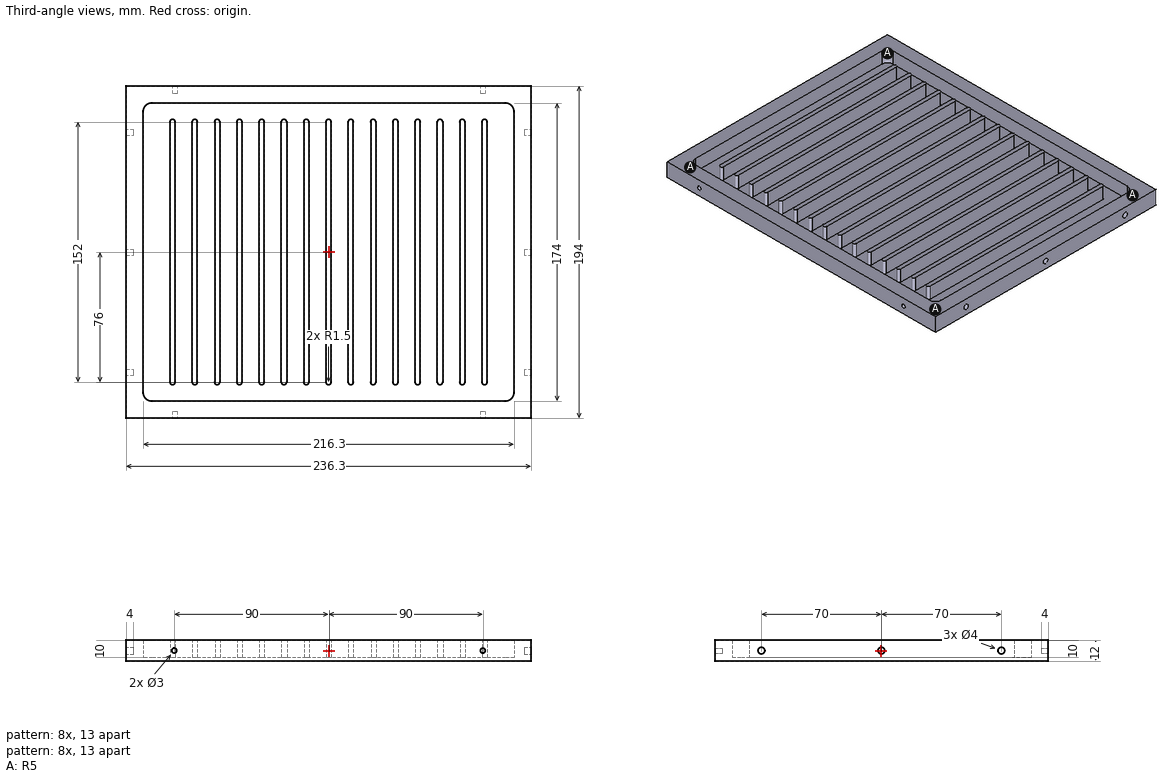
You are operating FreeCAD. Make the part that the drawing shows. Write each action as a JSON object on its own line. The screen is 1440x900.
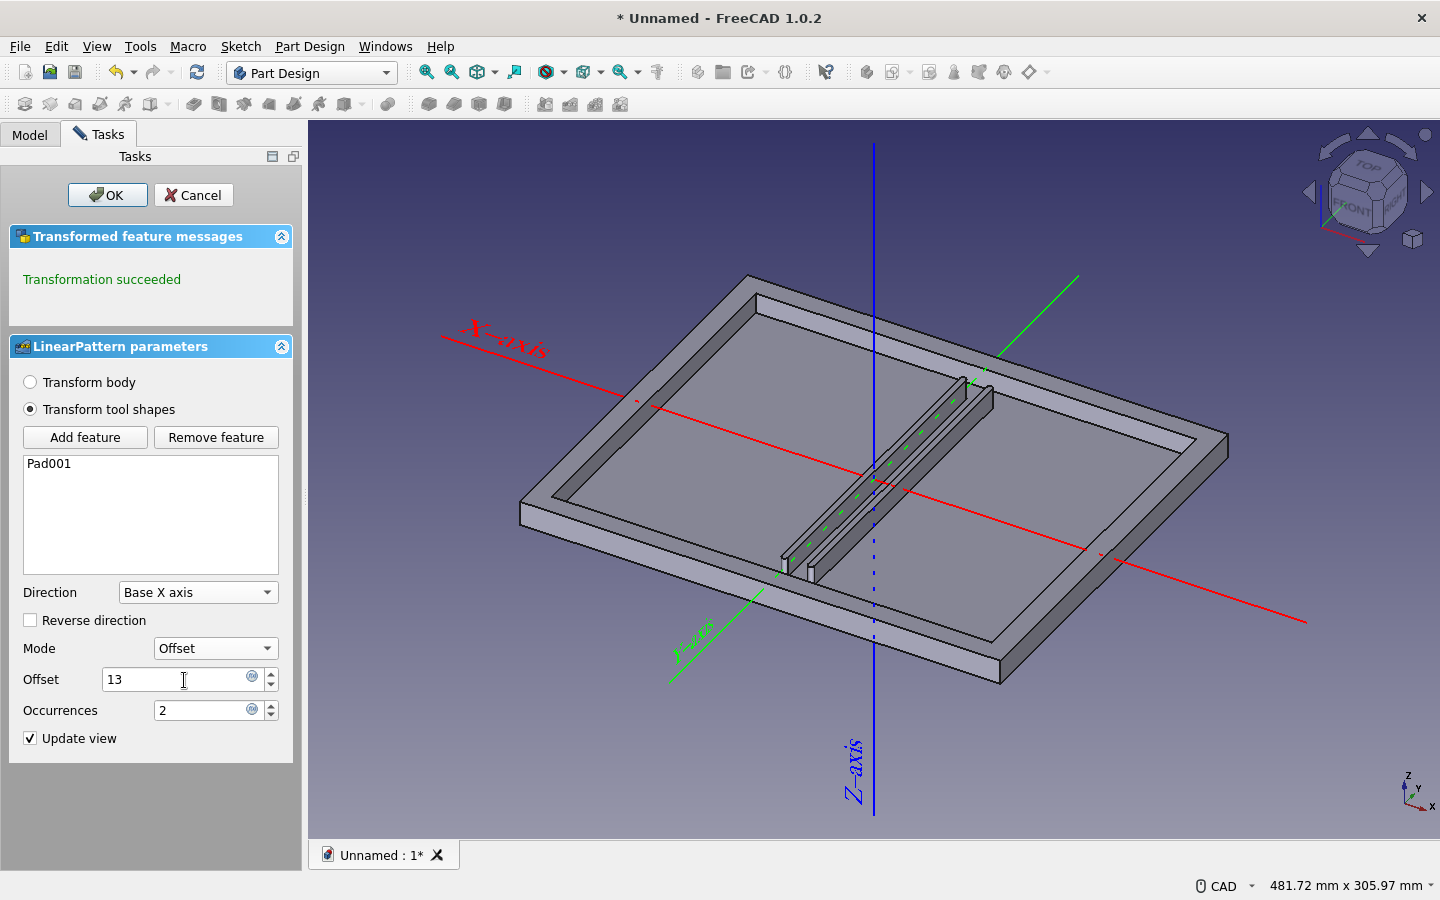
{"action": "triple_click", "coordinate": [210, 710]}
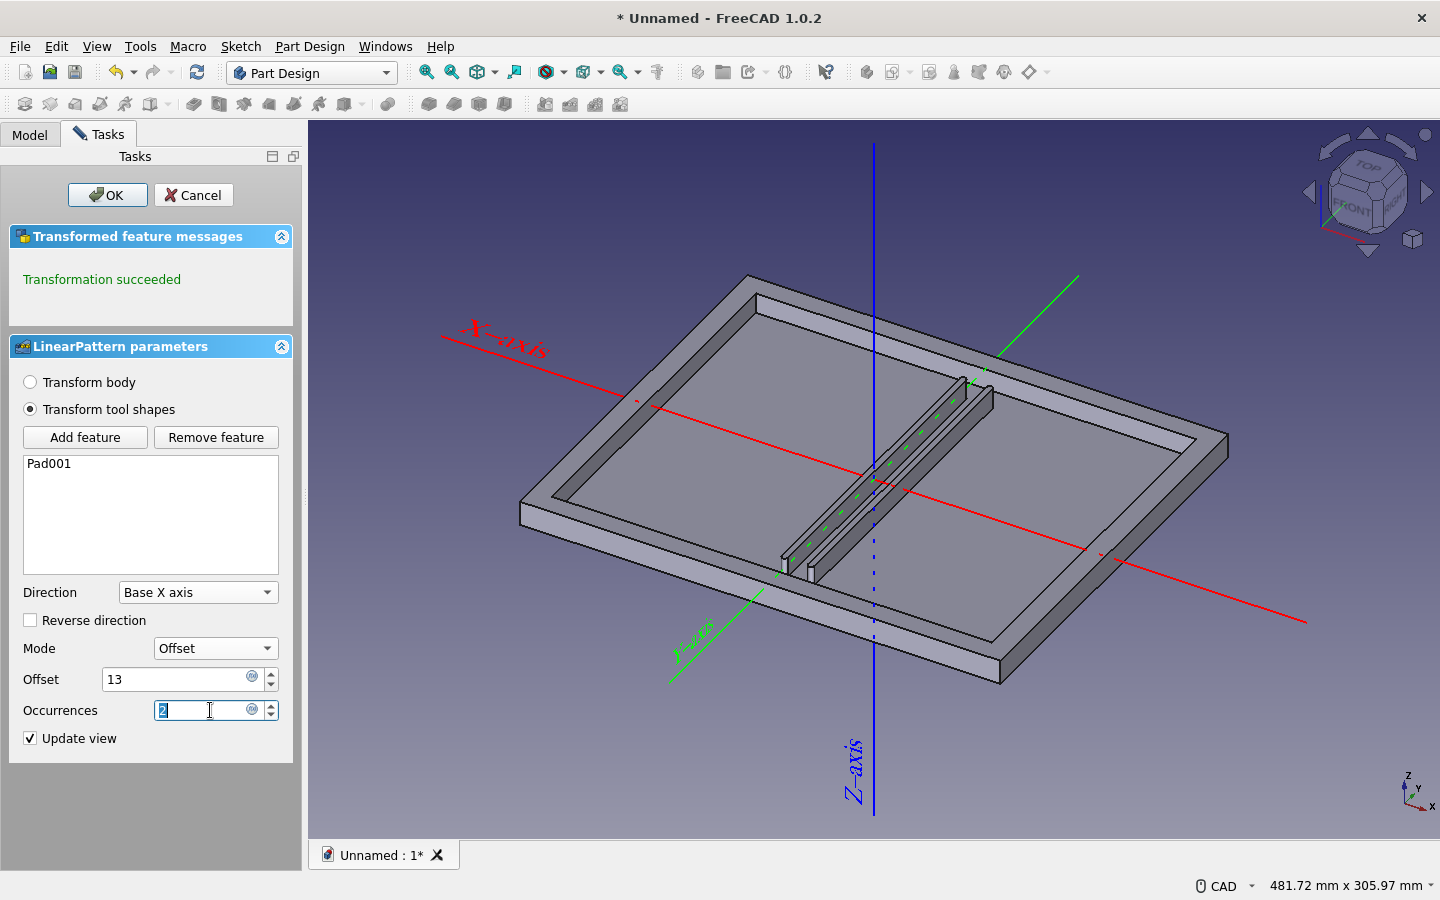
{"action": "type", "text": "8"}
{"action": "key", "text": "Tab"}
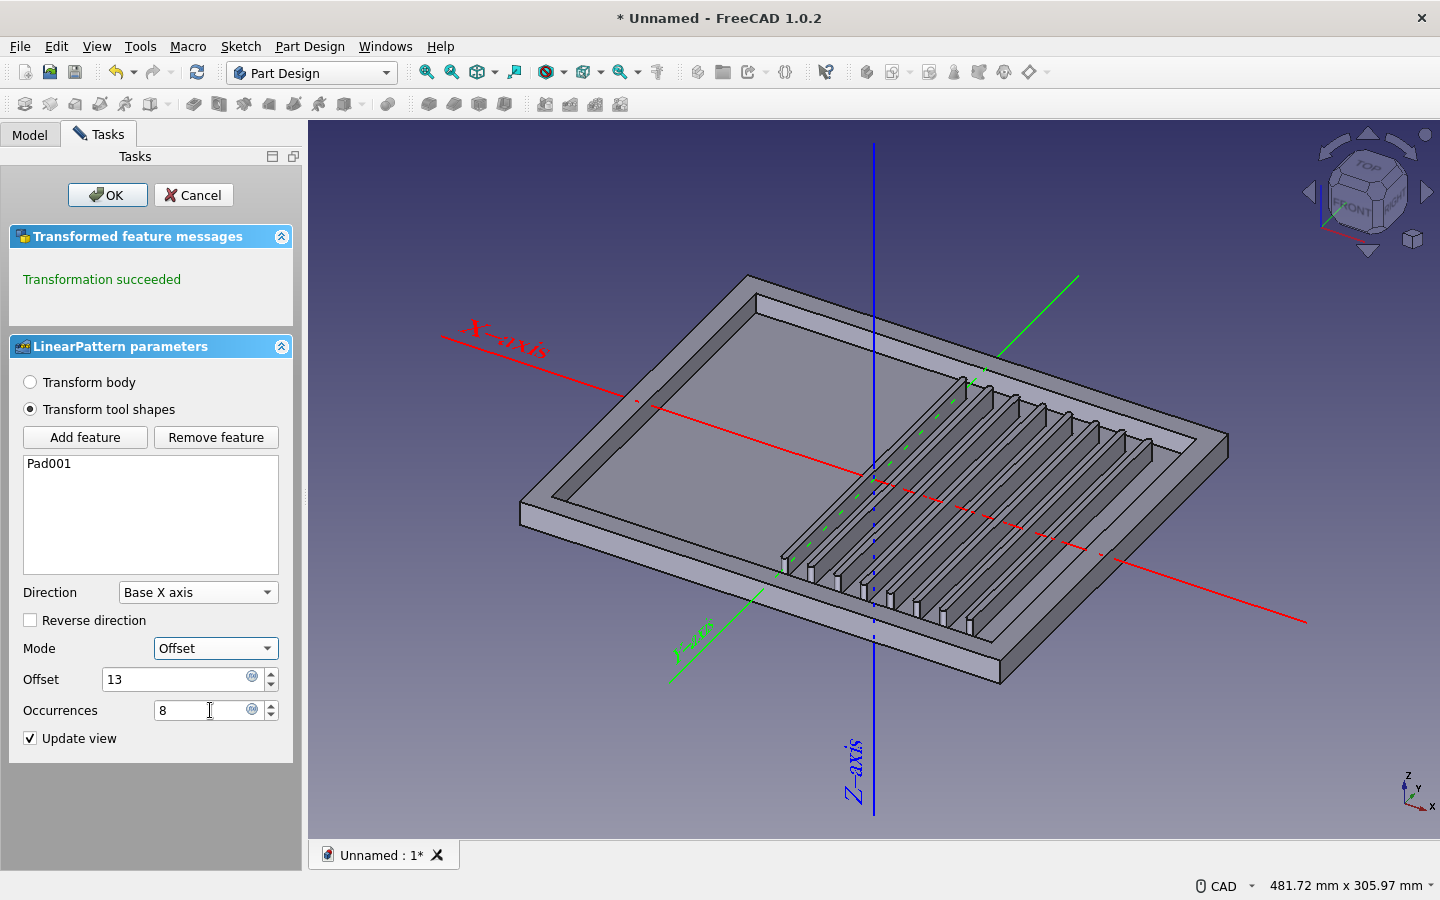
{"action": "left_click", "coordinate": [108, 195]}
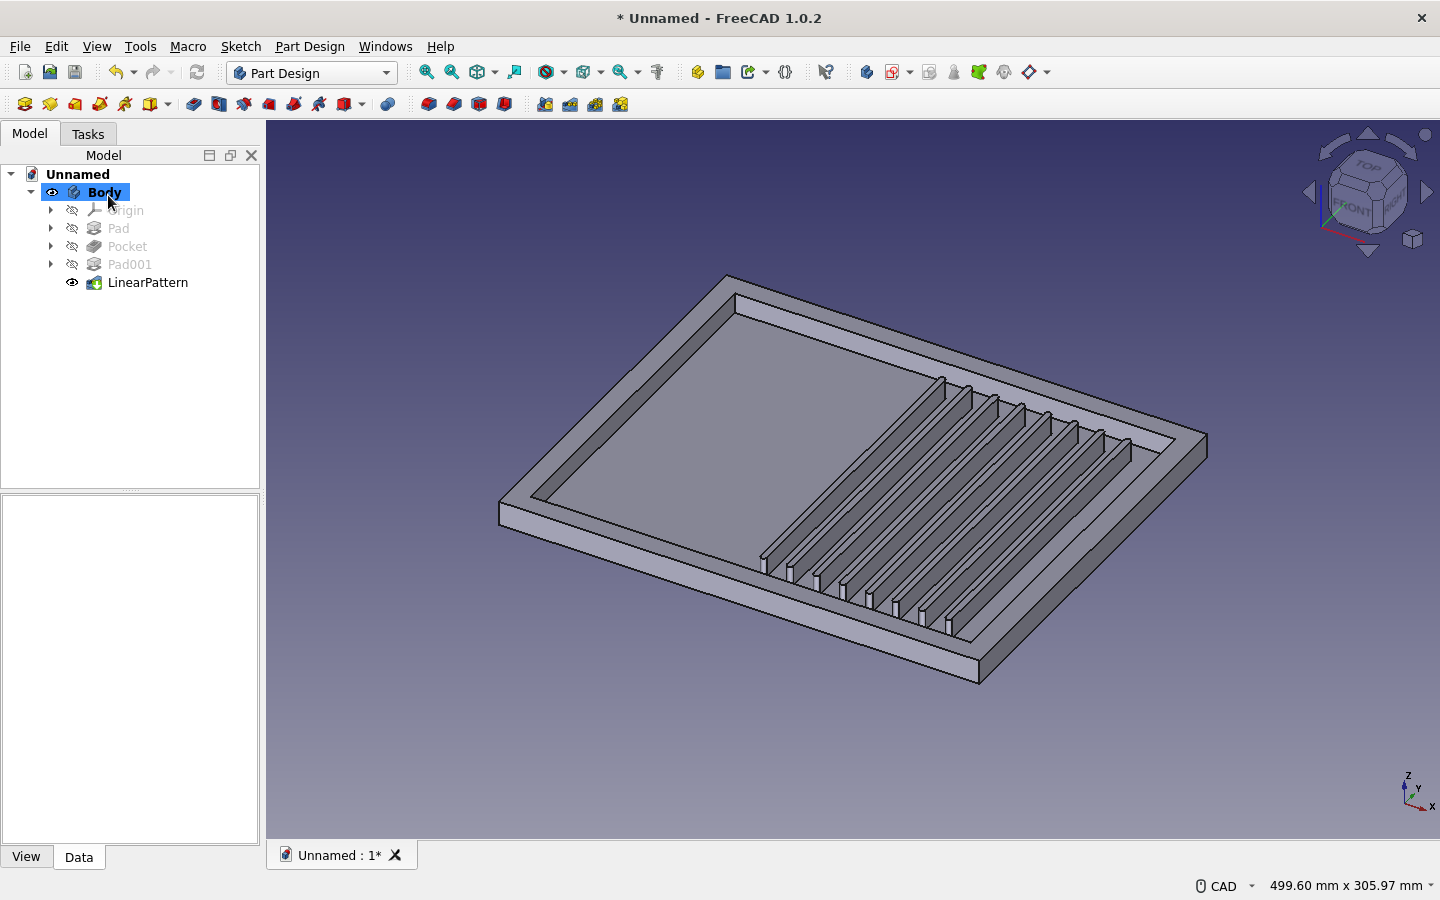
{"action": "left_click", "coordinate": [117, 264]}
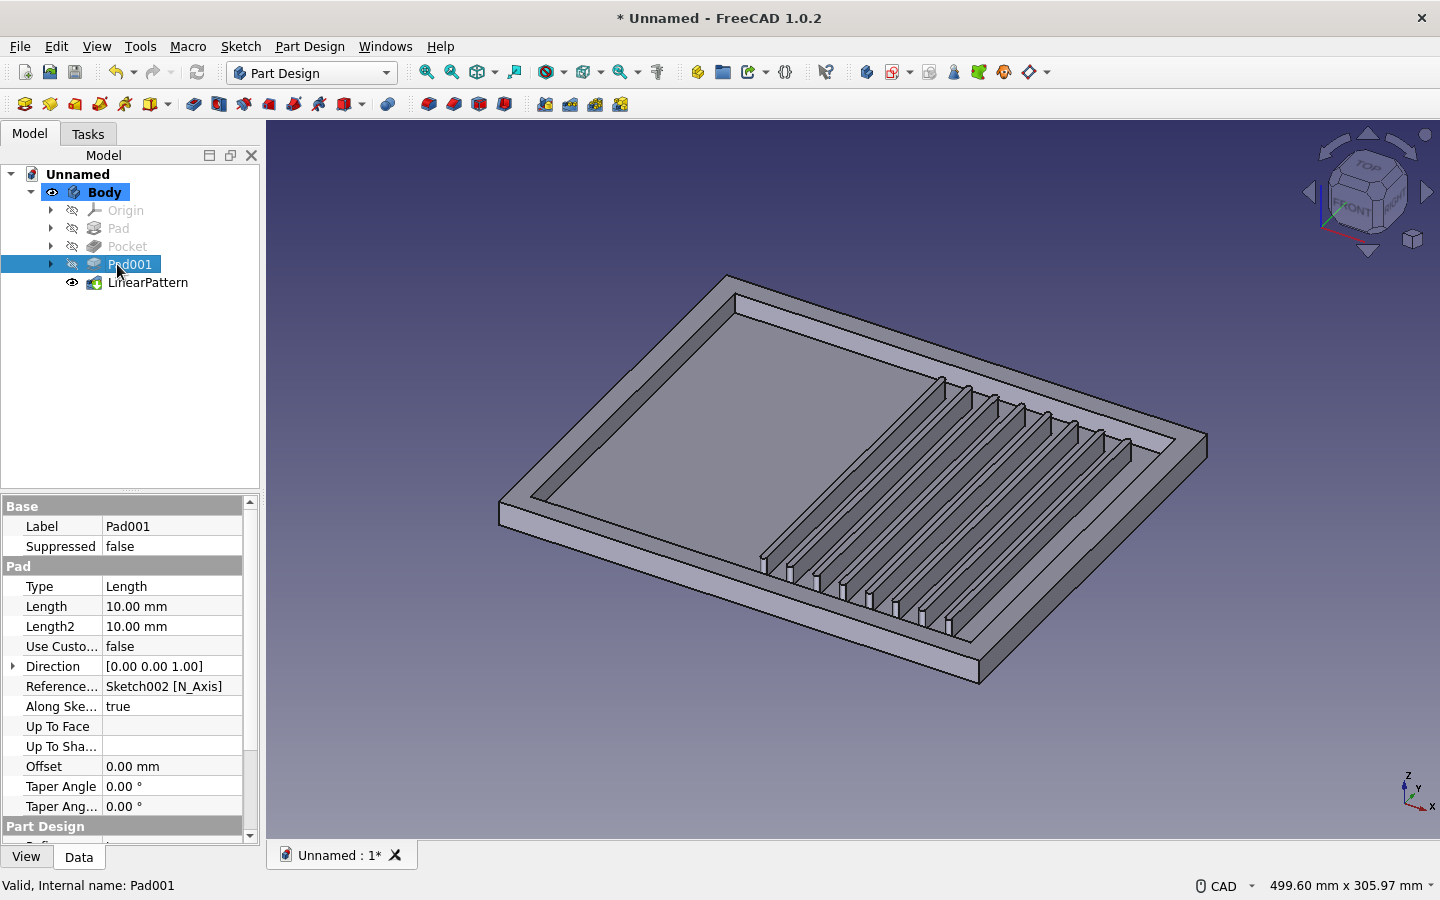
{"action": "left_click", "coordinate": [570, 104]}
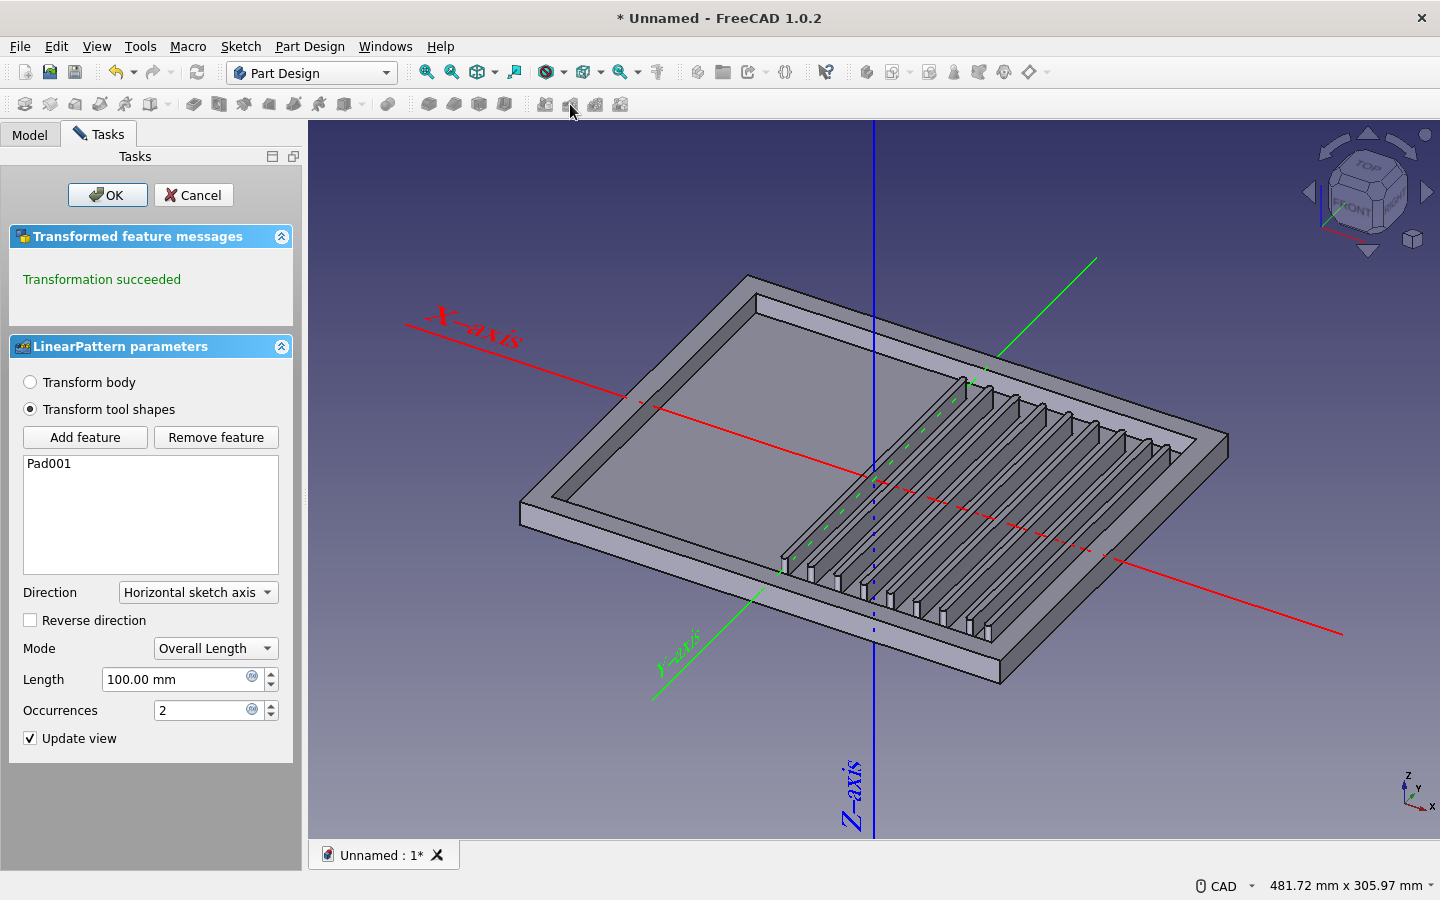
{"action": "left_click", "coordinate": [199, 592]}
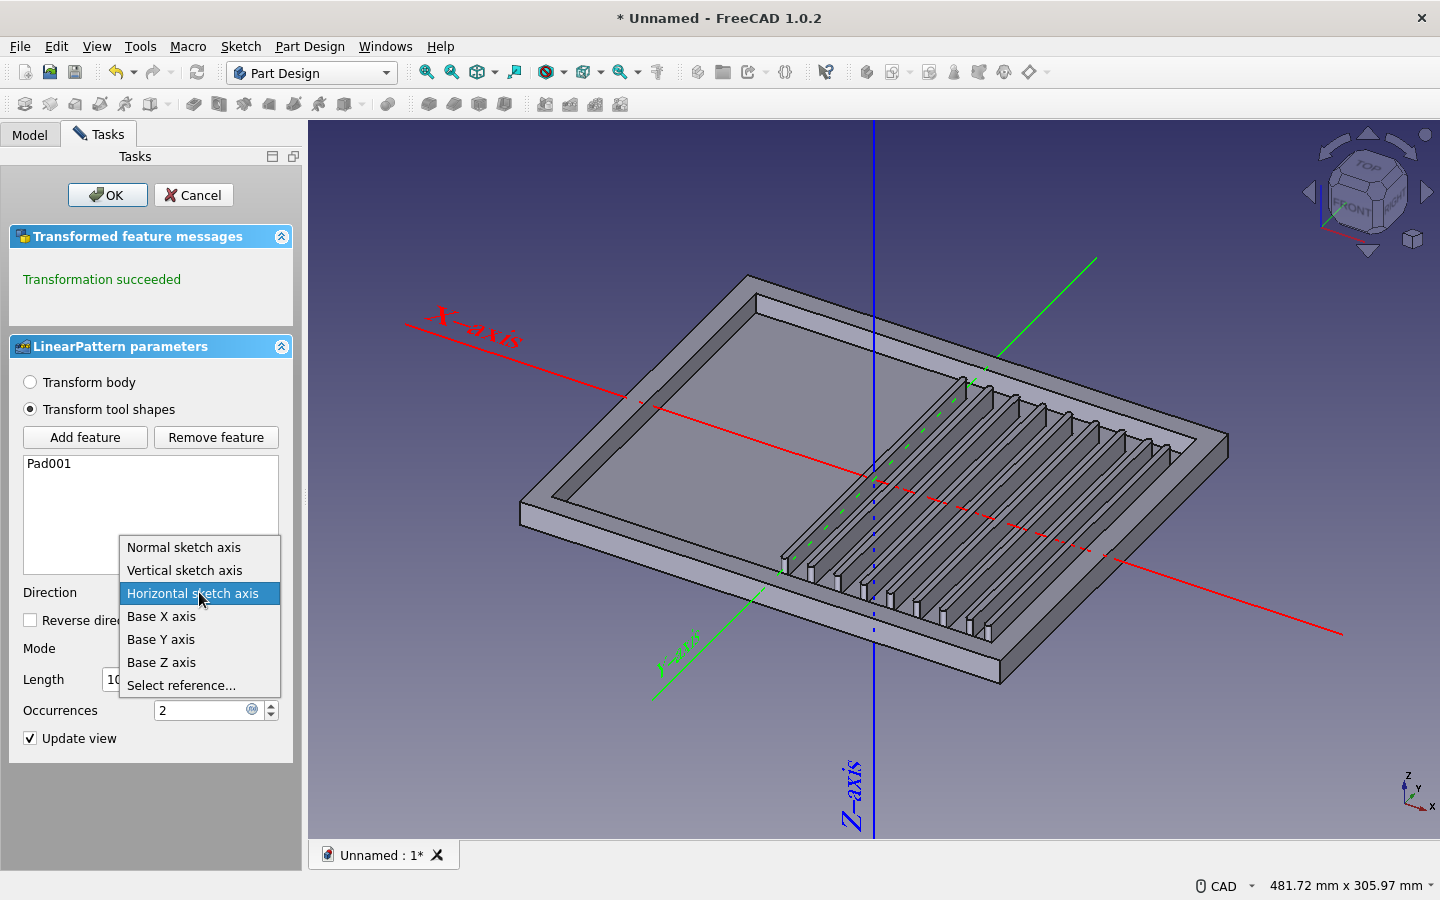
{"action": "left_click", "coordinate": [198, 616]}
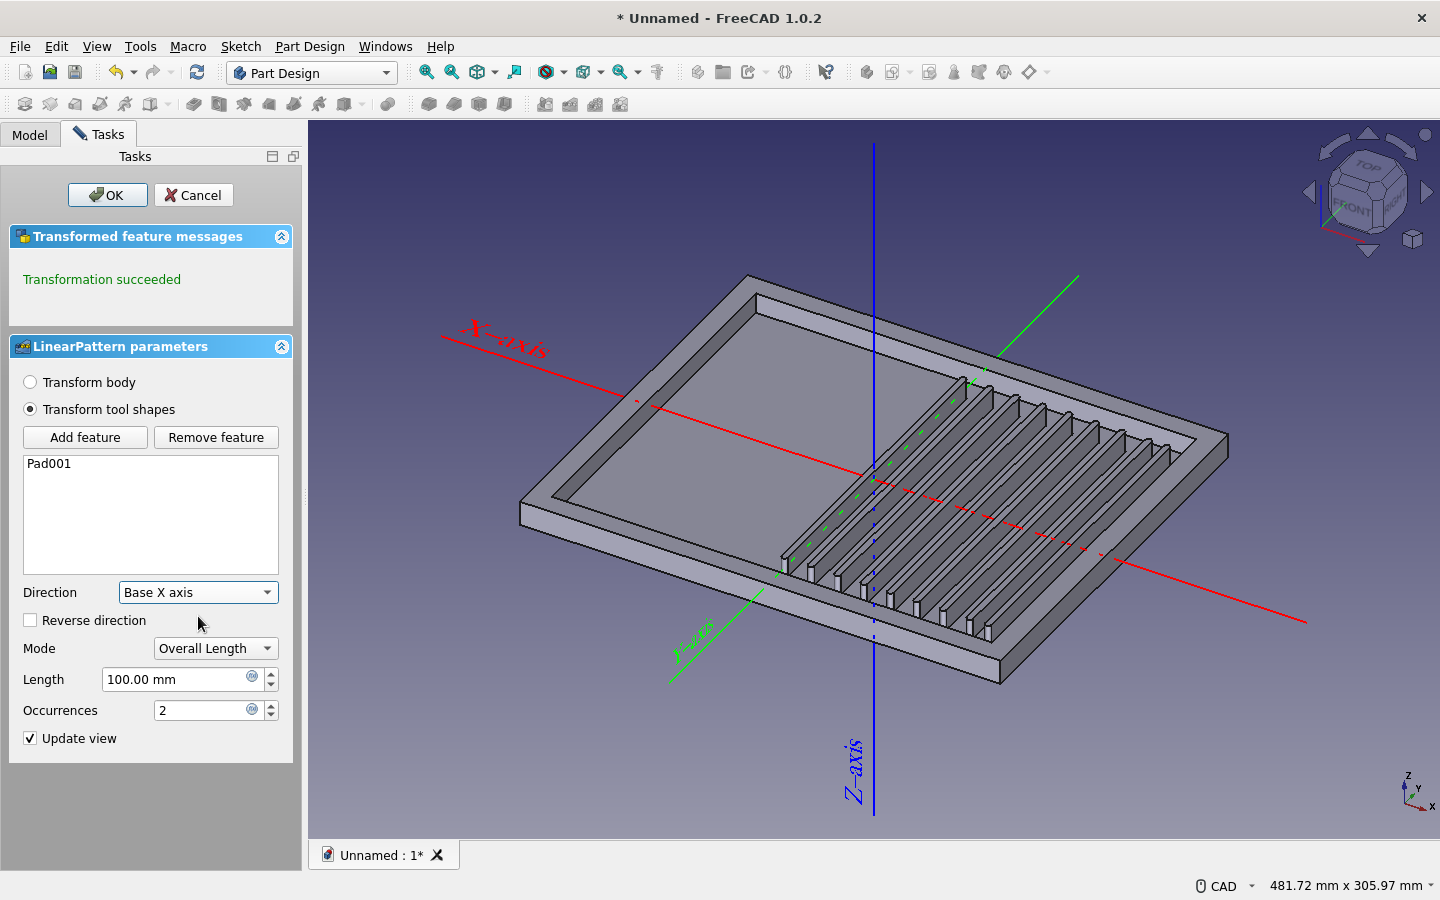
{"action": "left_click", "coordinate": [216, 648]}